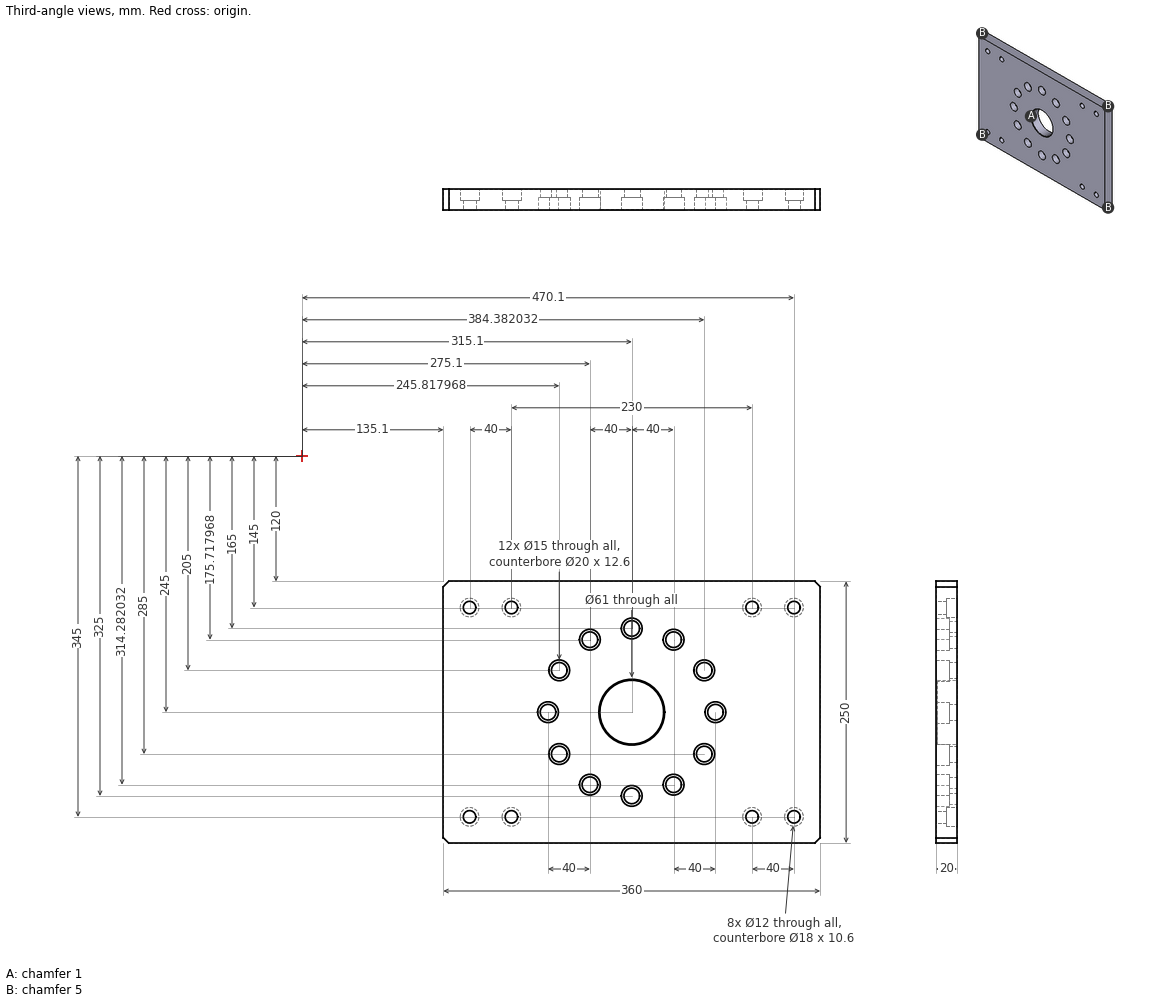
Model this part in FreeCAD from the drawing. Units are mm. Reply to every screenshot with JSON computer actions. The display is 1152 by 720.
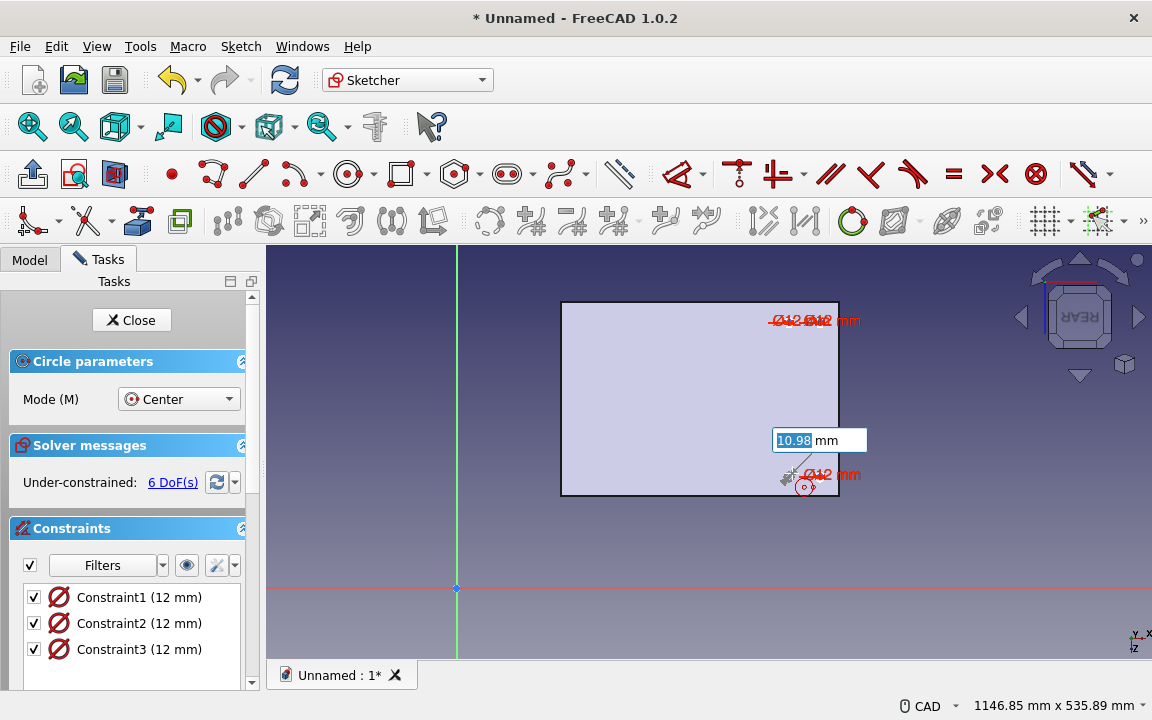
{"action": "type", "text": "12"}
{"action": "key", "text": "Return"}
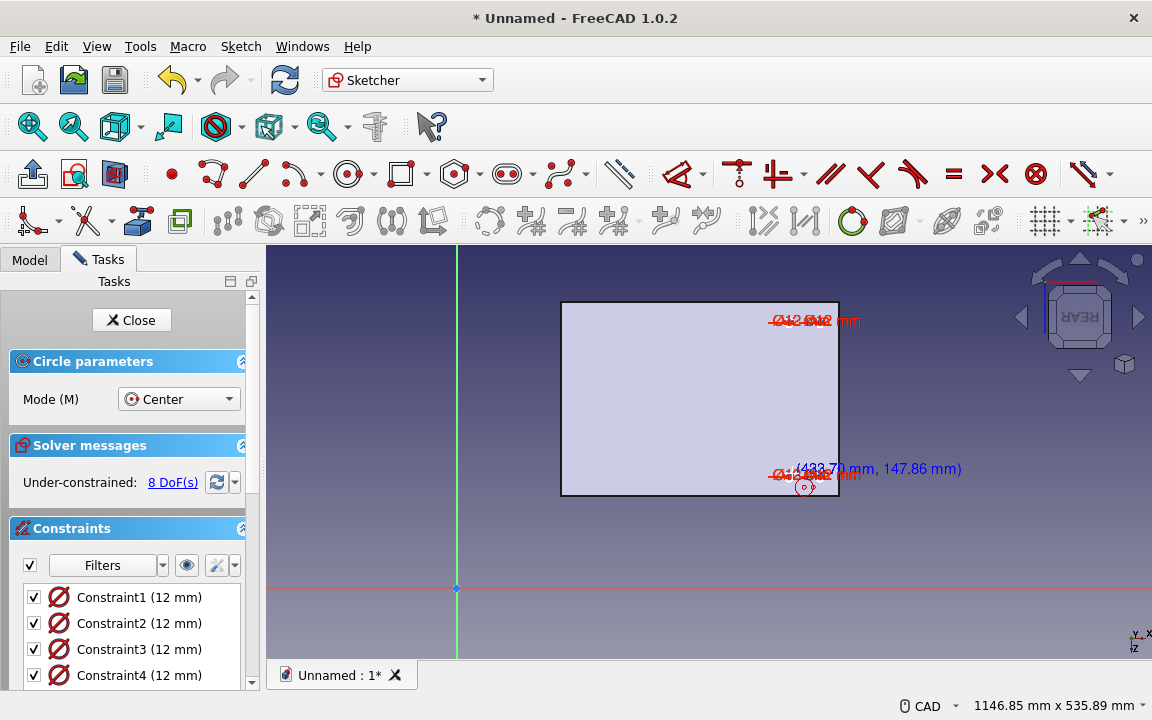
{"action": "scroll", "coordinate": [612, 476], "scroll_direction": "up", "scroll_amount": 8}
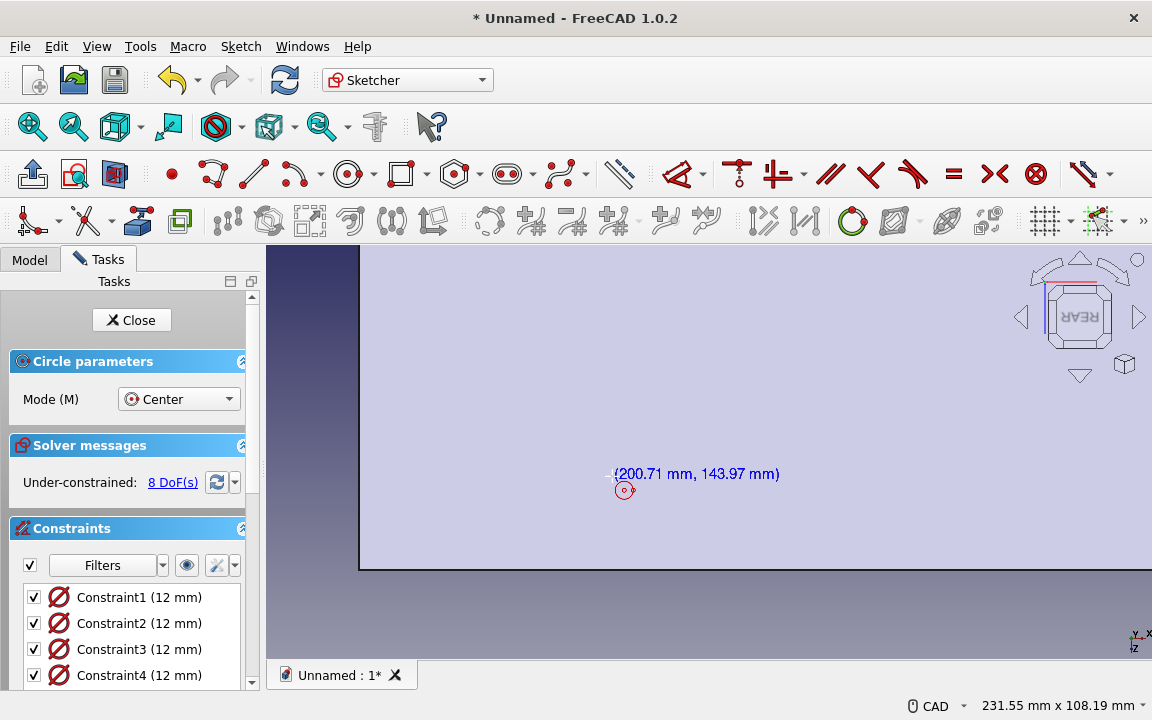
{"action": "scroll", "coordinate": [612, 476], "scroll_direction": "down", "scroll_amount": 8}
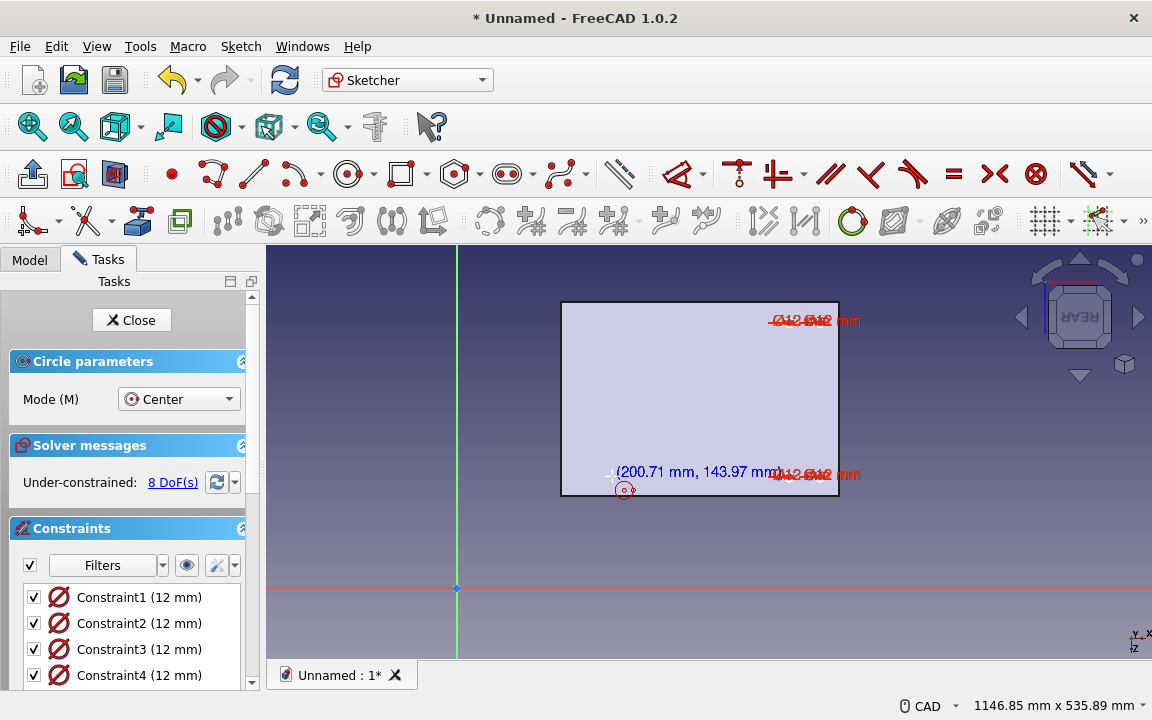
{"action": "left_click", "coordinate": [612, 476]}
{"action": "mouse_move", "coordinate": [615, 473]}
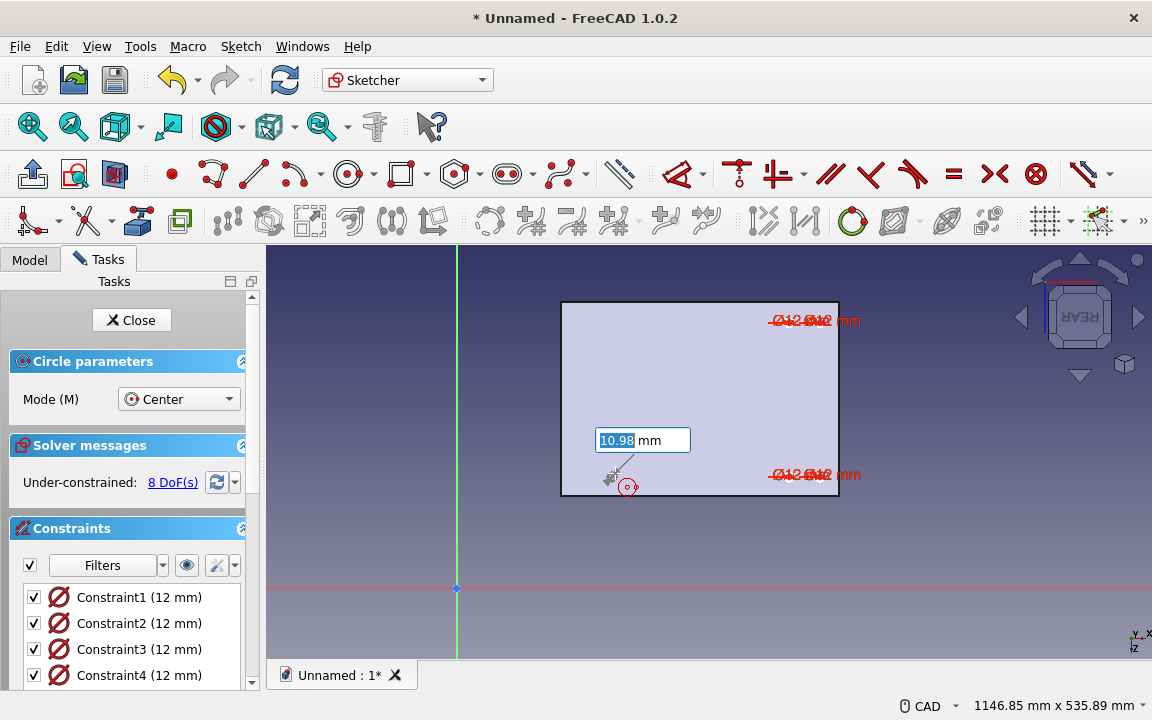
{"action": "type", "text": "12"}
{"action": "key", "text": "Return"}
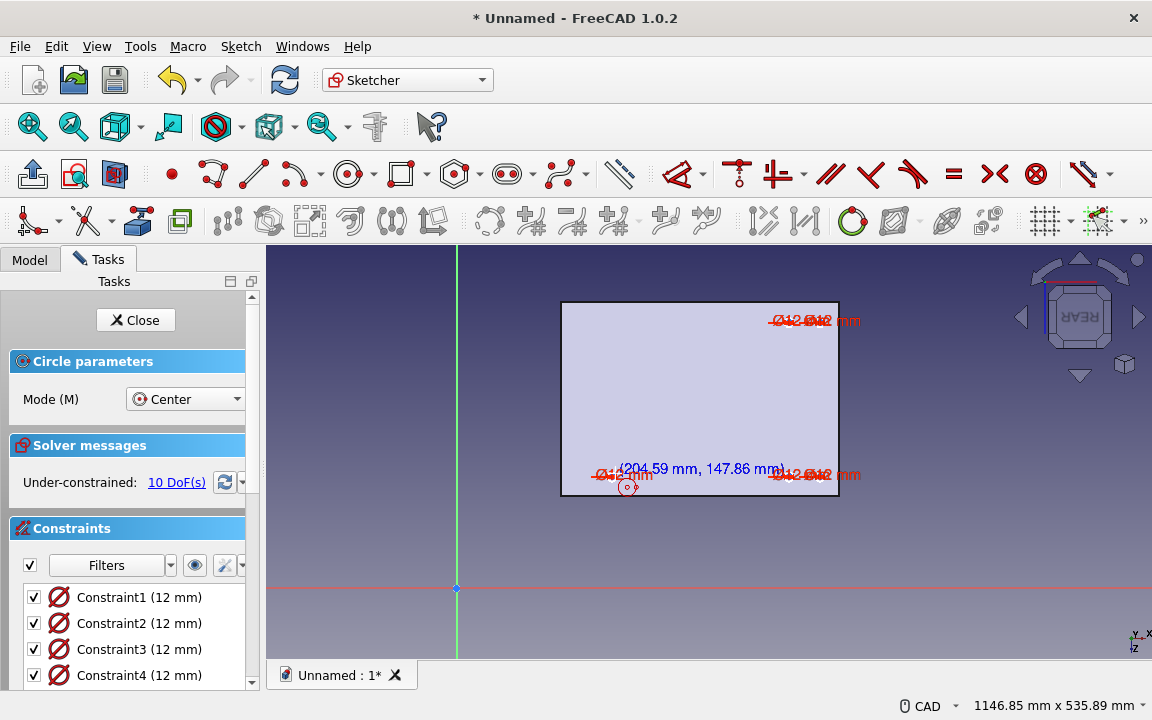
{"action": "scroll", "coordinate": [612, 322], "scroll_direction": "up", "scroll_amount": 8}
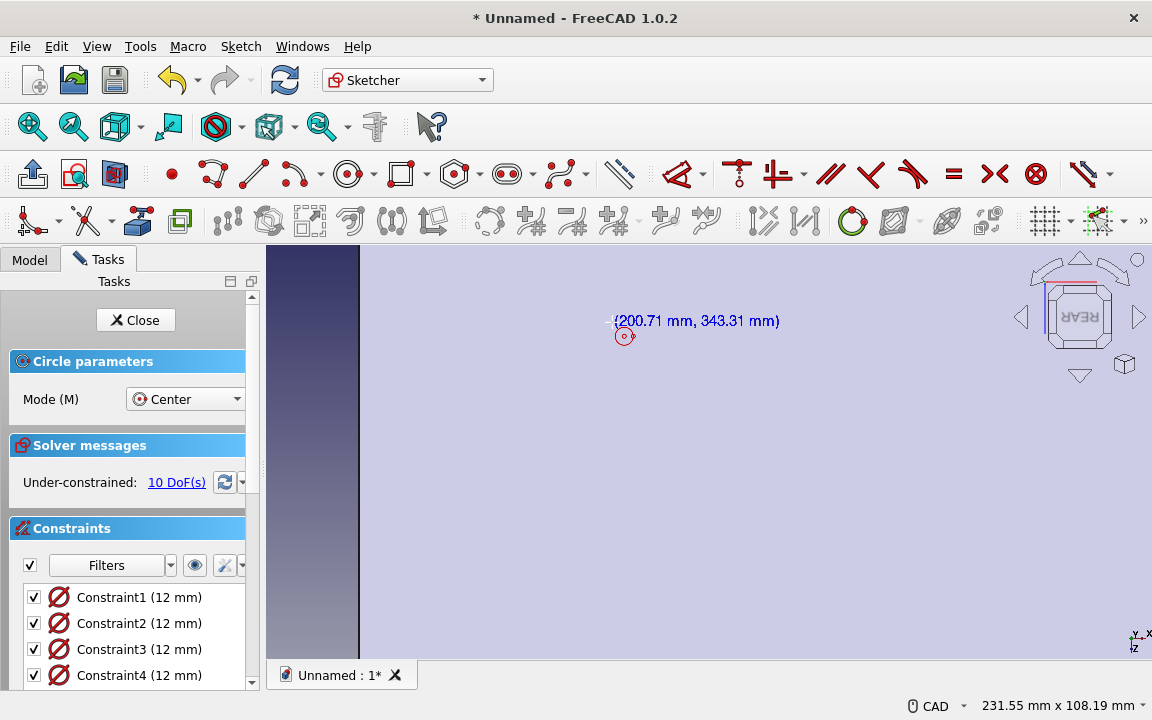
{"action": "scroll", "coordinate": [612, 321], "scroll_direction": "down", "scroll_amount": 8}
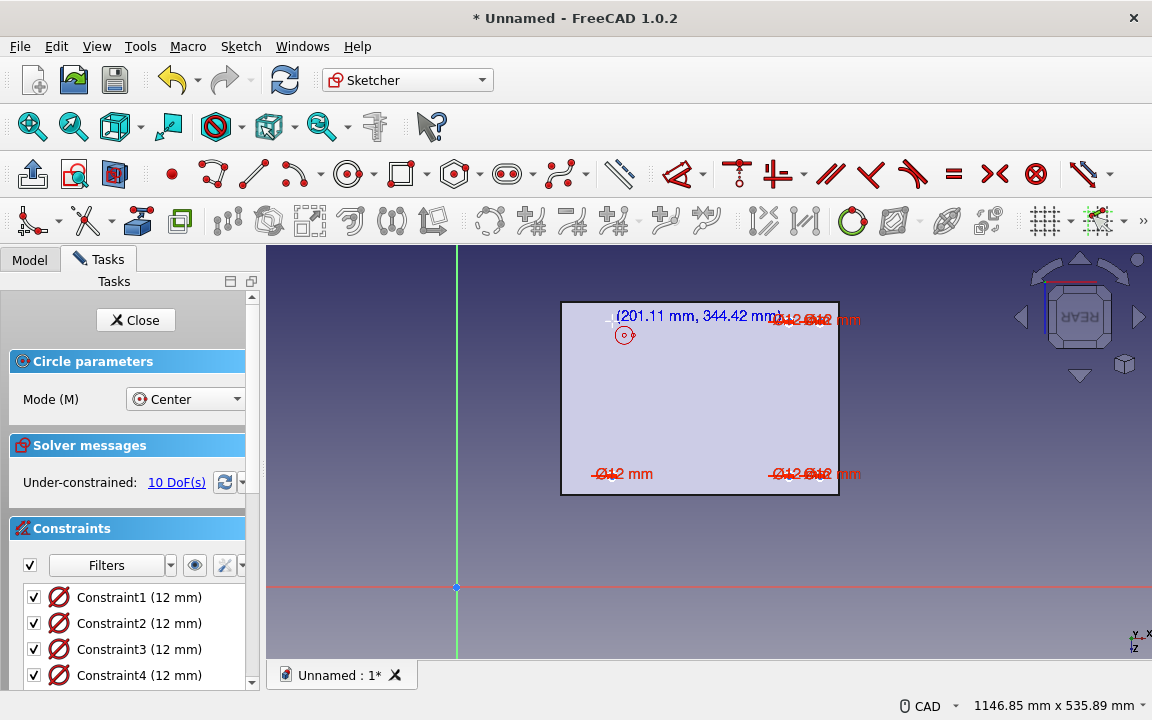
{"action": "left_click", "coordinate": [612, 321]}
{"action": "mouse_move", "coordinate": [615, 318]}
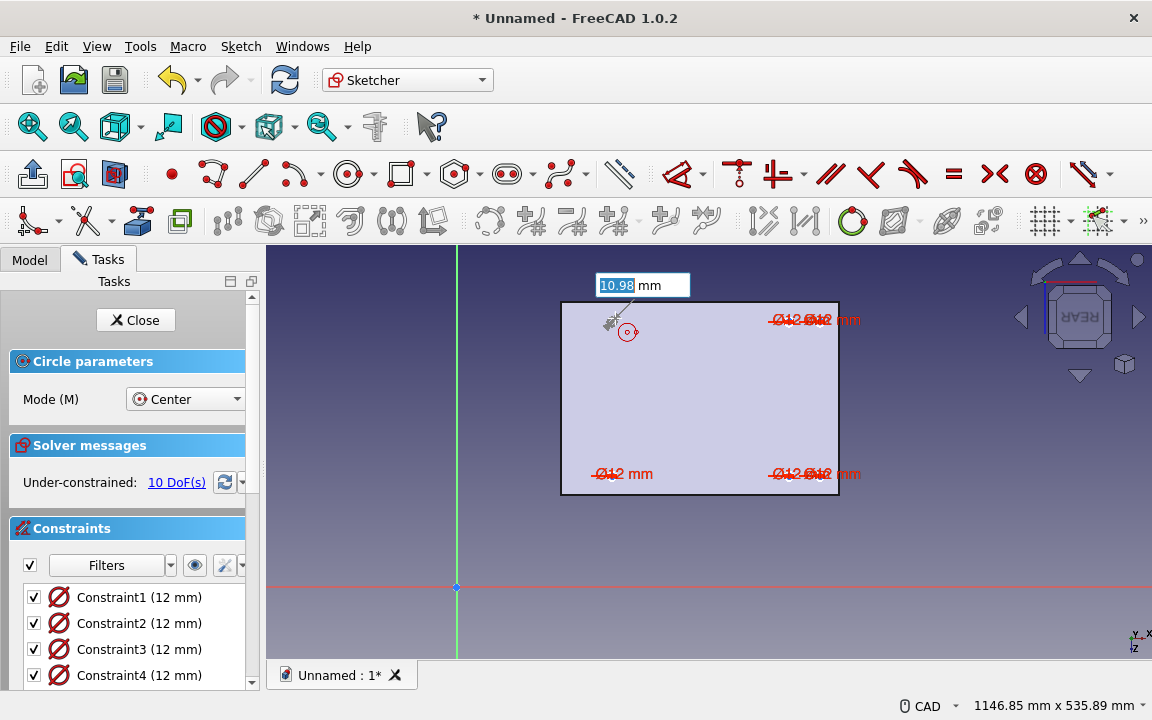
{"action": "type", "text": "12"}
{"action": "key", "text": "Return"}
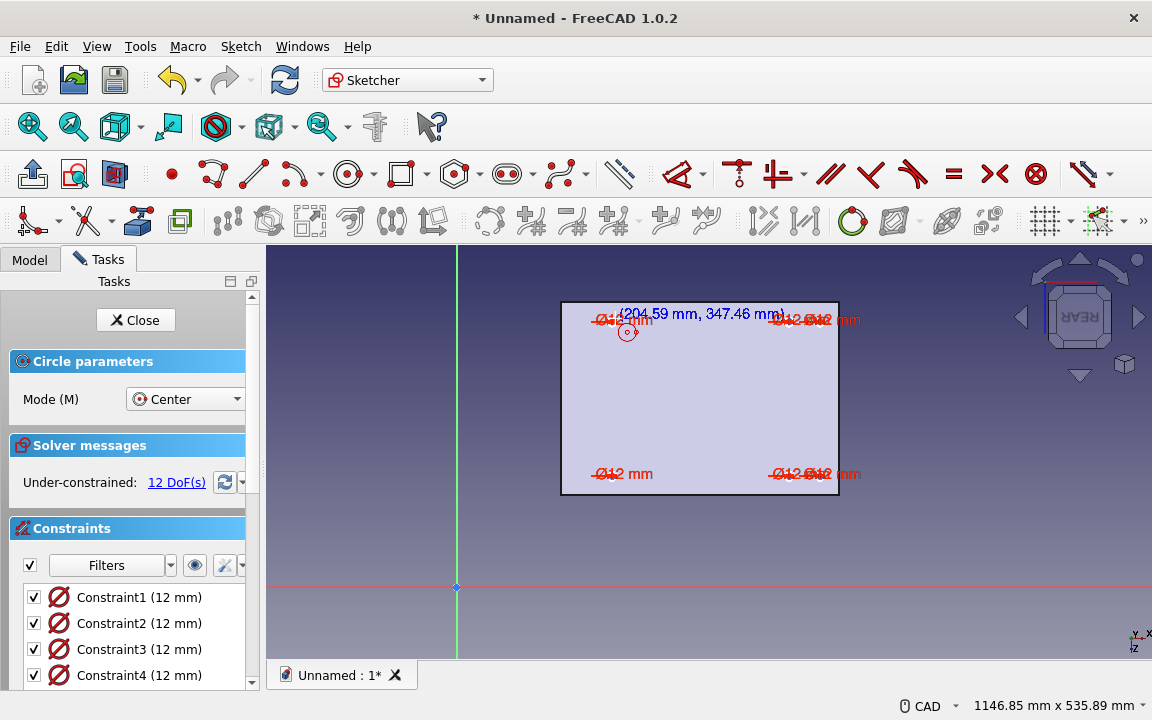
{"action": "scroll", "coordinate": [581, 475], "scroll_direction": "up", "scroll_amount": 8}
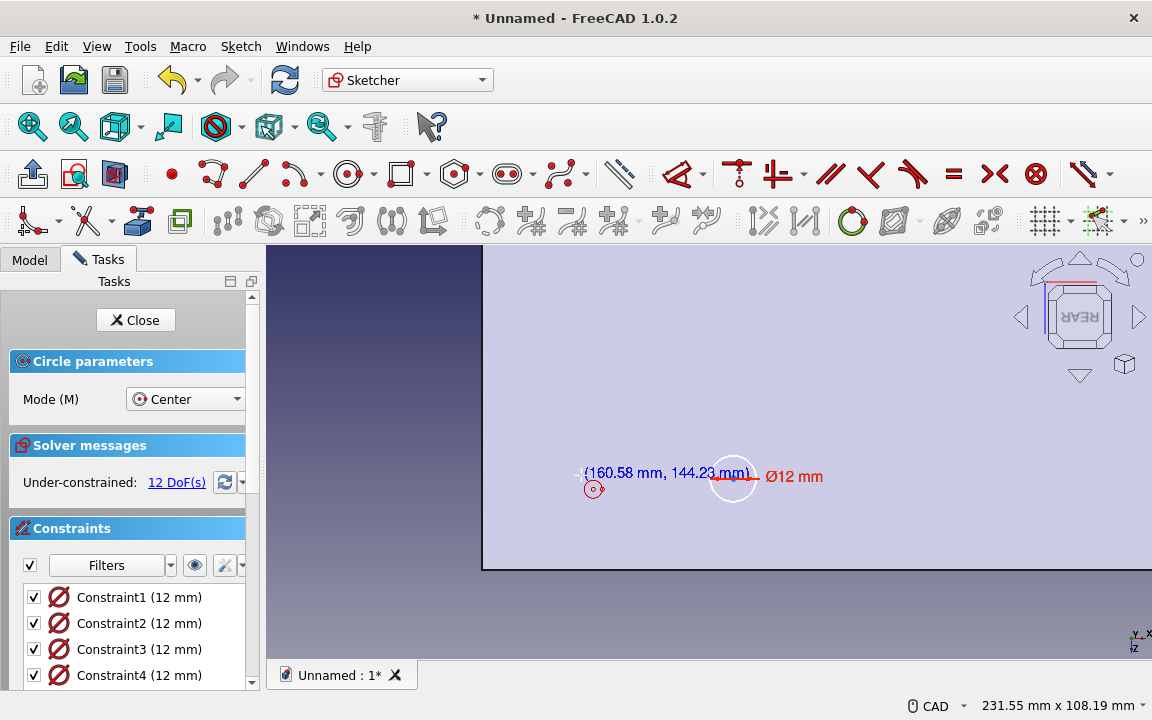
{"action": "scroll", "coordinate": [581, 476], "scroll_direction": "down", "scroll_amount": 8}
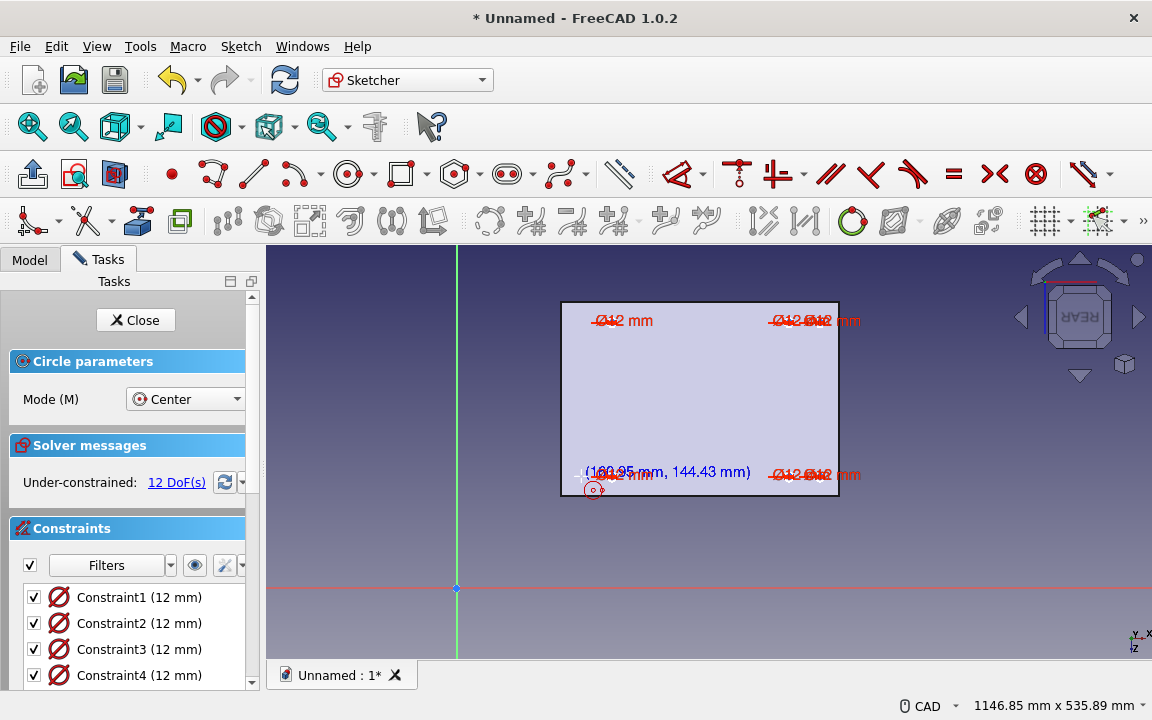
{"action": "left_click", "coordinate": [581, 476]}
{"action": "mouse_move", "coordinate": [584, 473]}